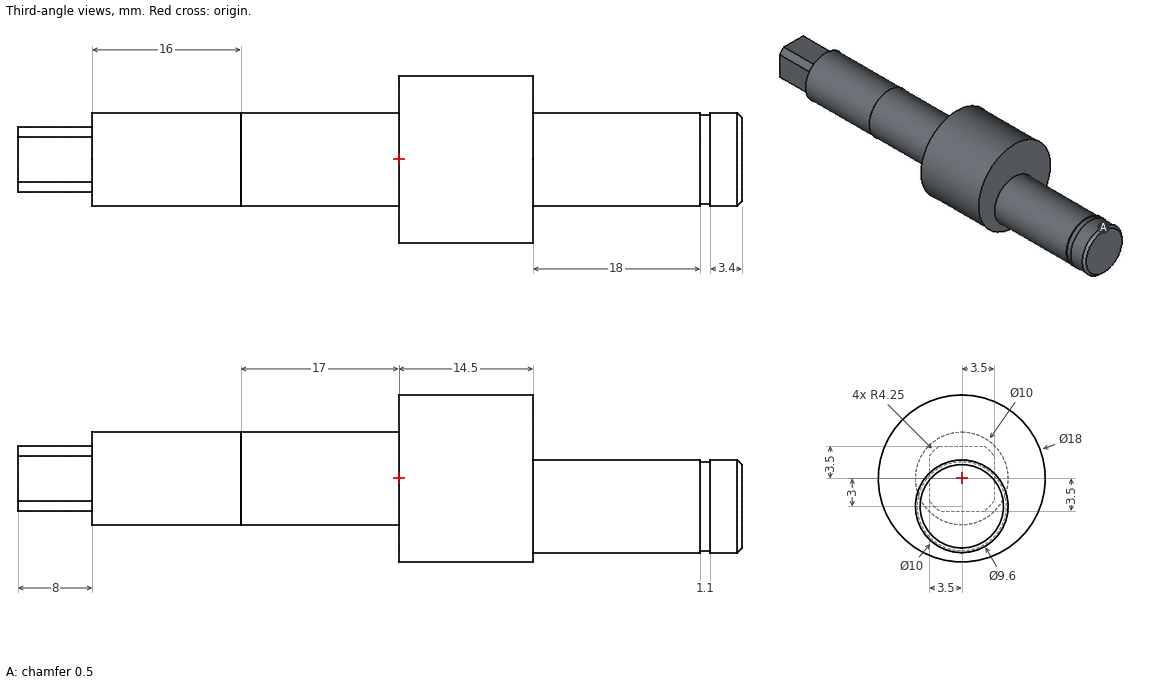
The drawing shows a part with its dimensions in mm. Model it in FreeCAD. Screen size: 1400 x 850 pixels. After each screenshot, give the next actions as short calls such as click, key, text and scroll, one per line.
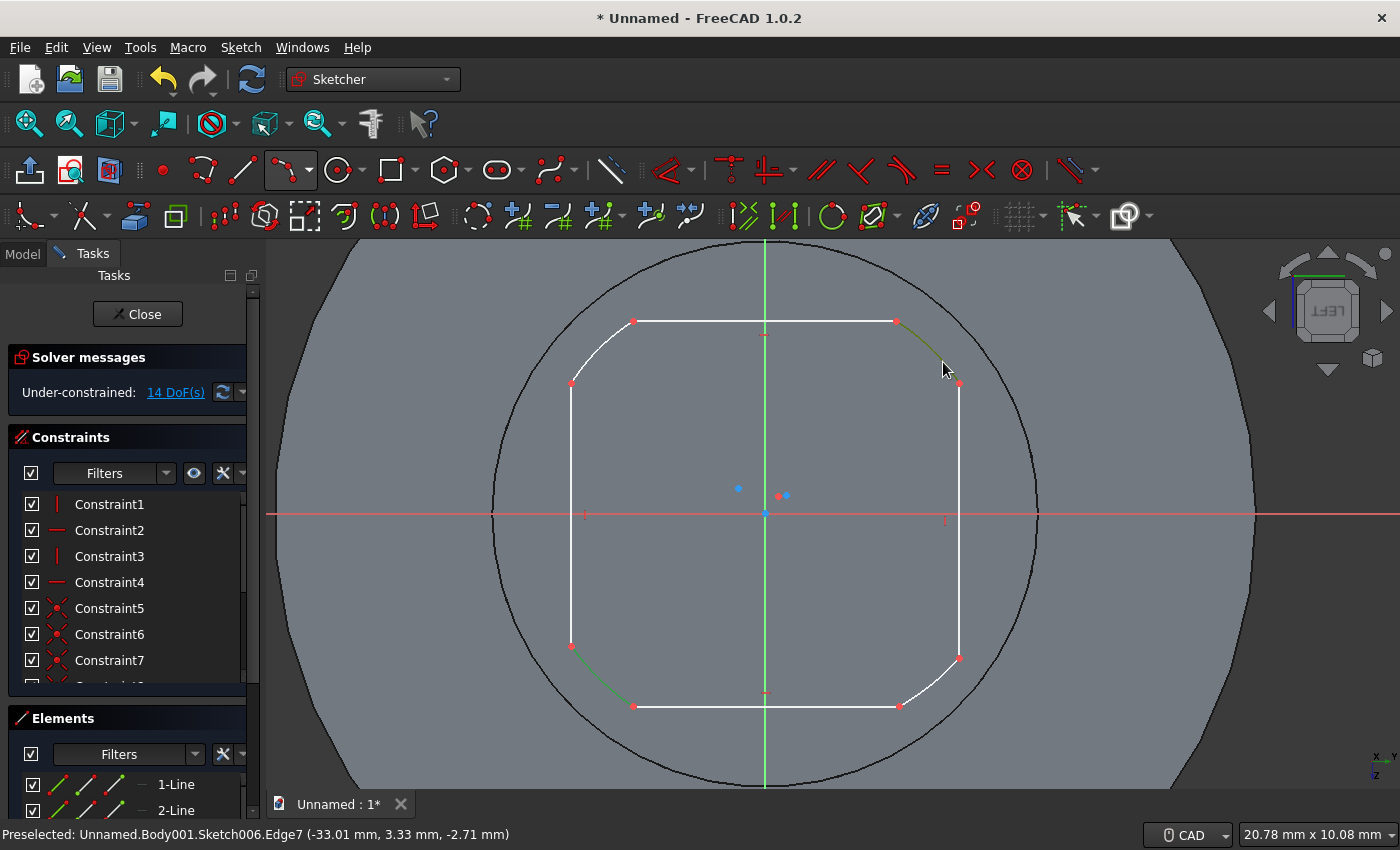
click(730, 170)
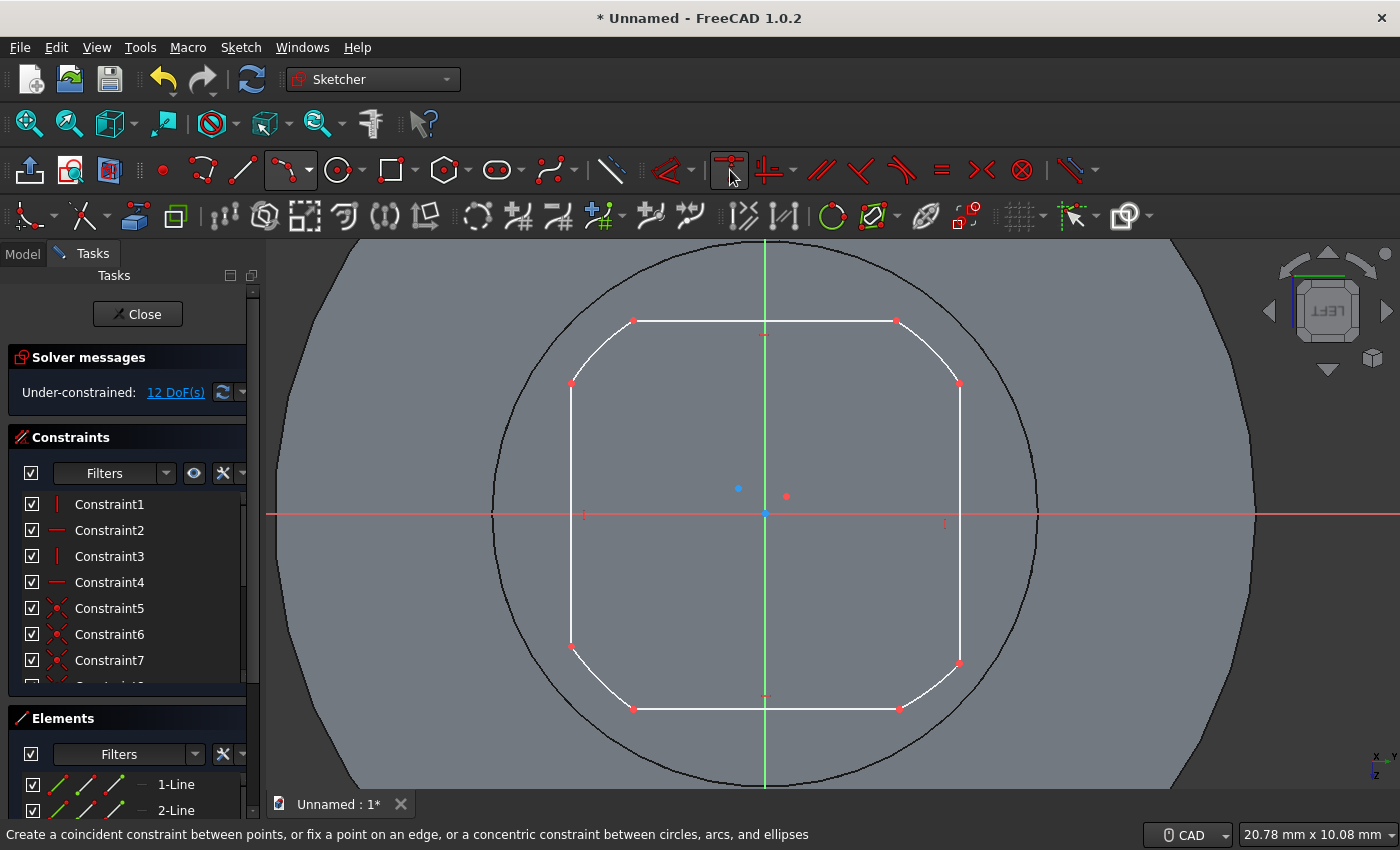
click(588, 667)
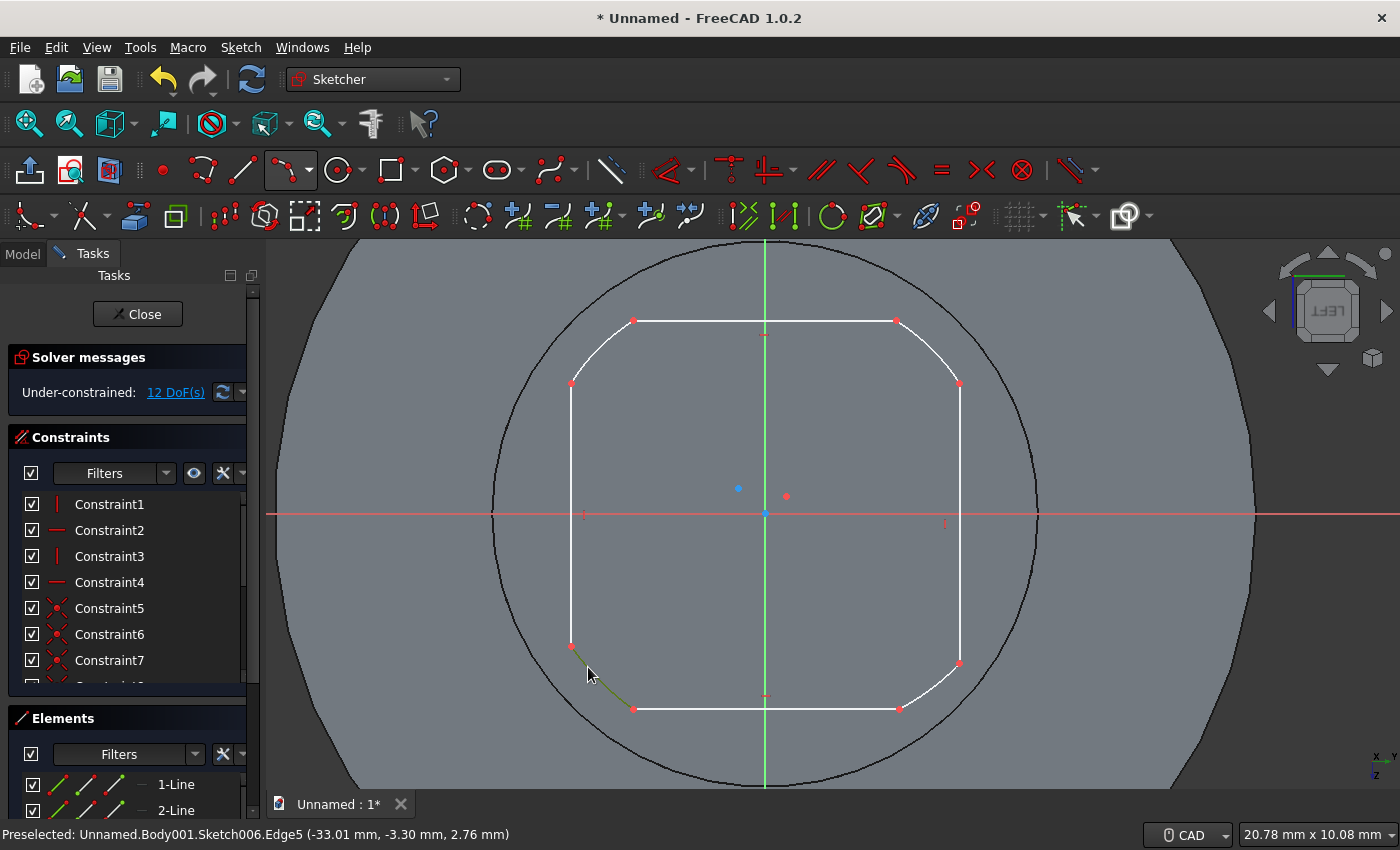
click(612, 337)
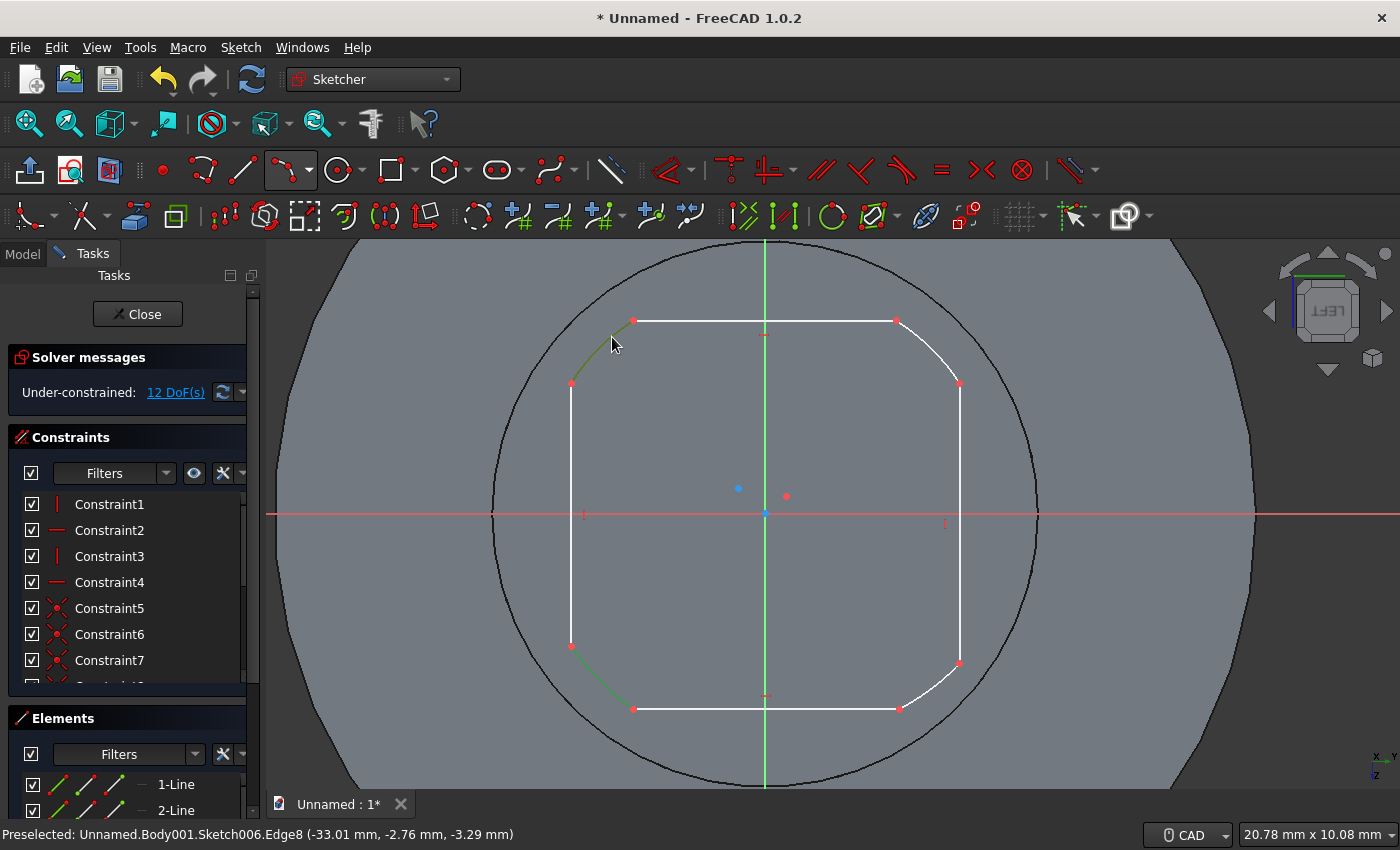
click(730, 170)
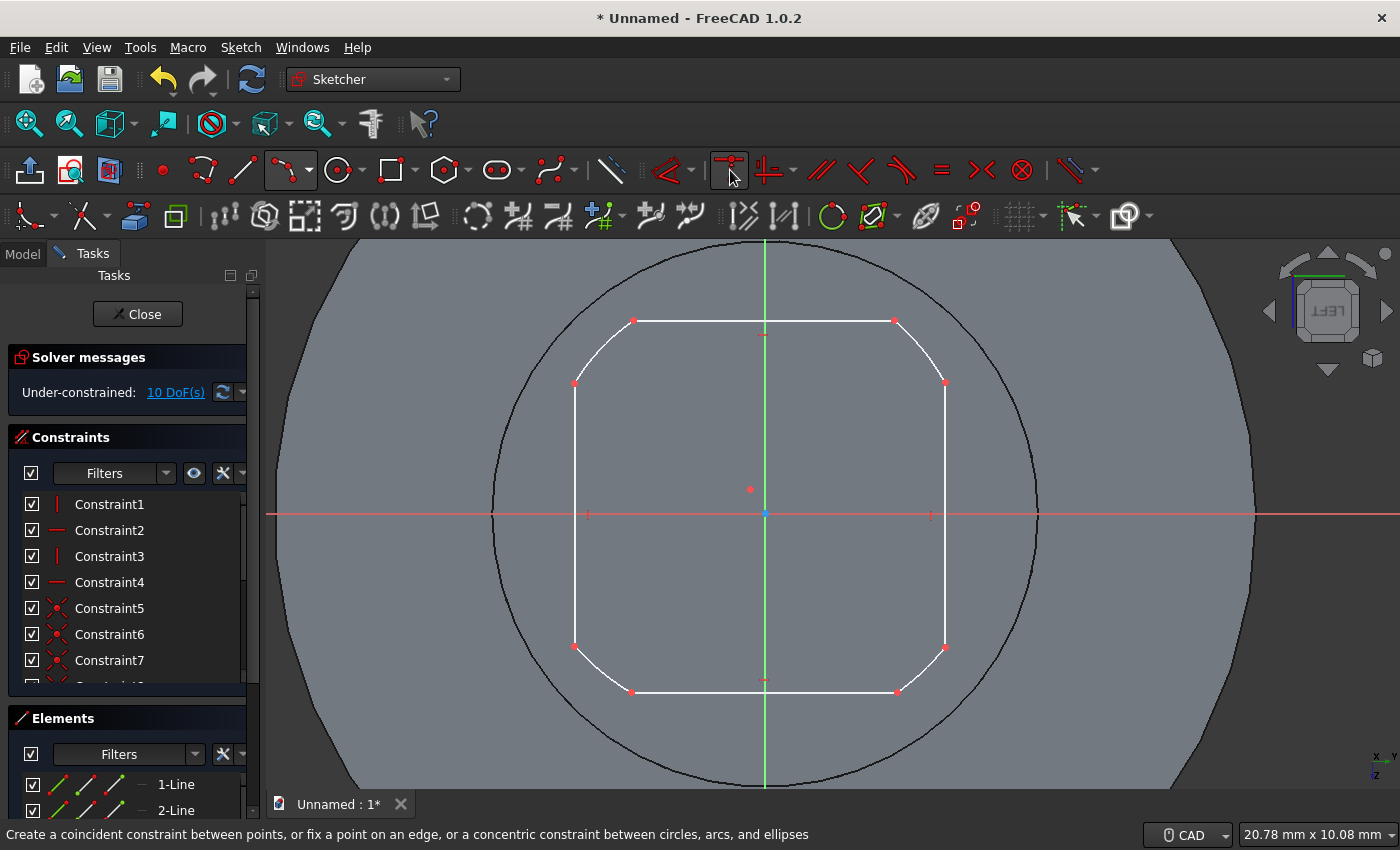
drag(741, 480, 775, 524)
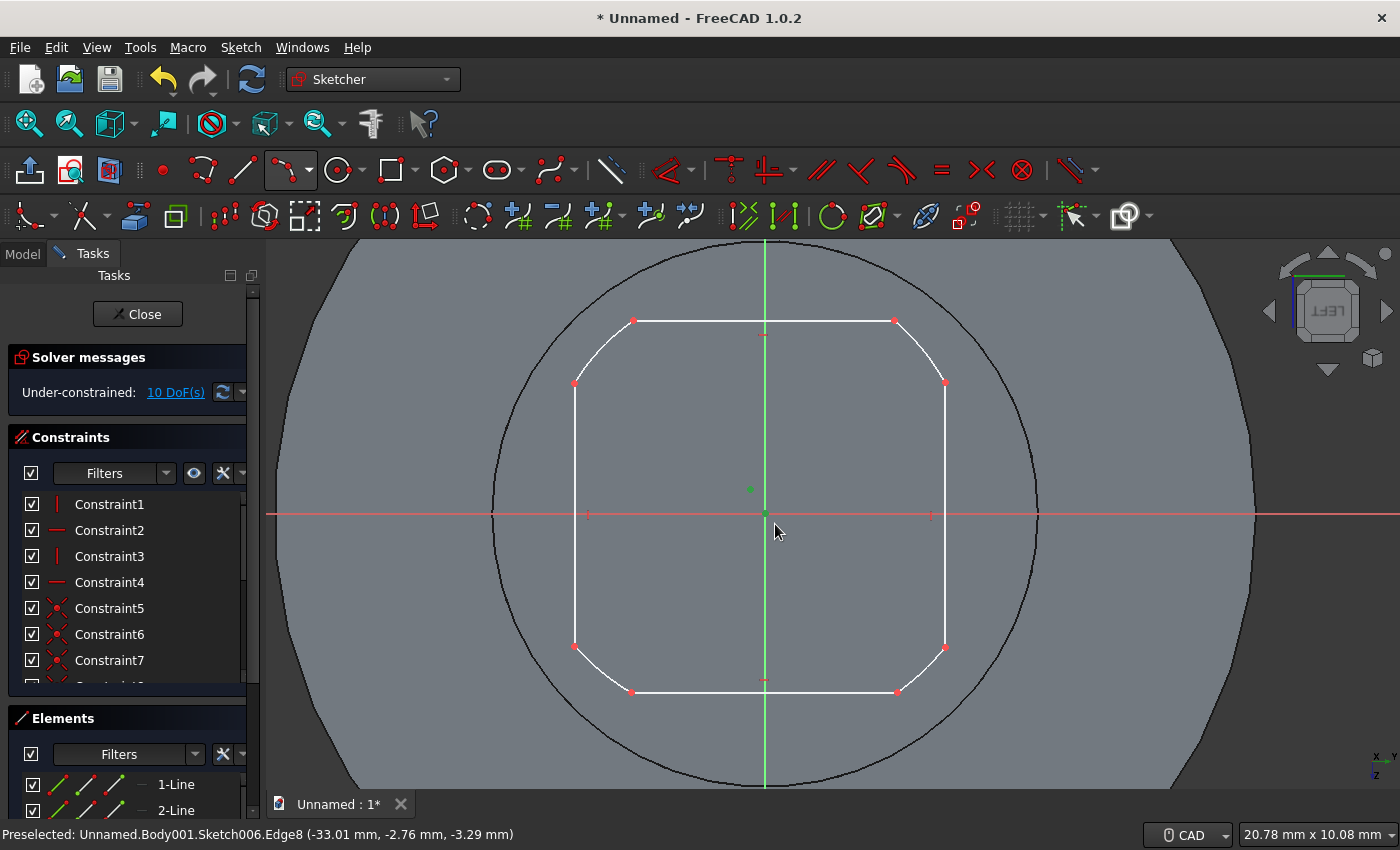
click(730, 170)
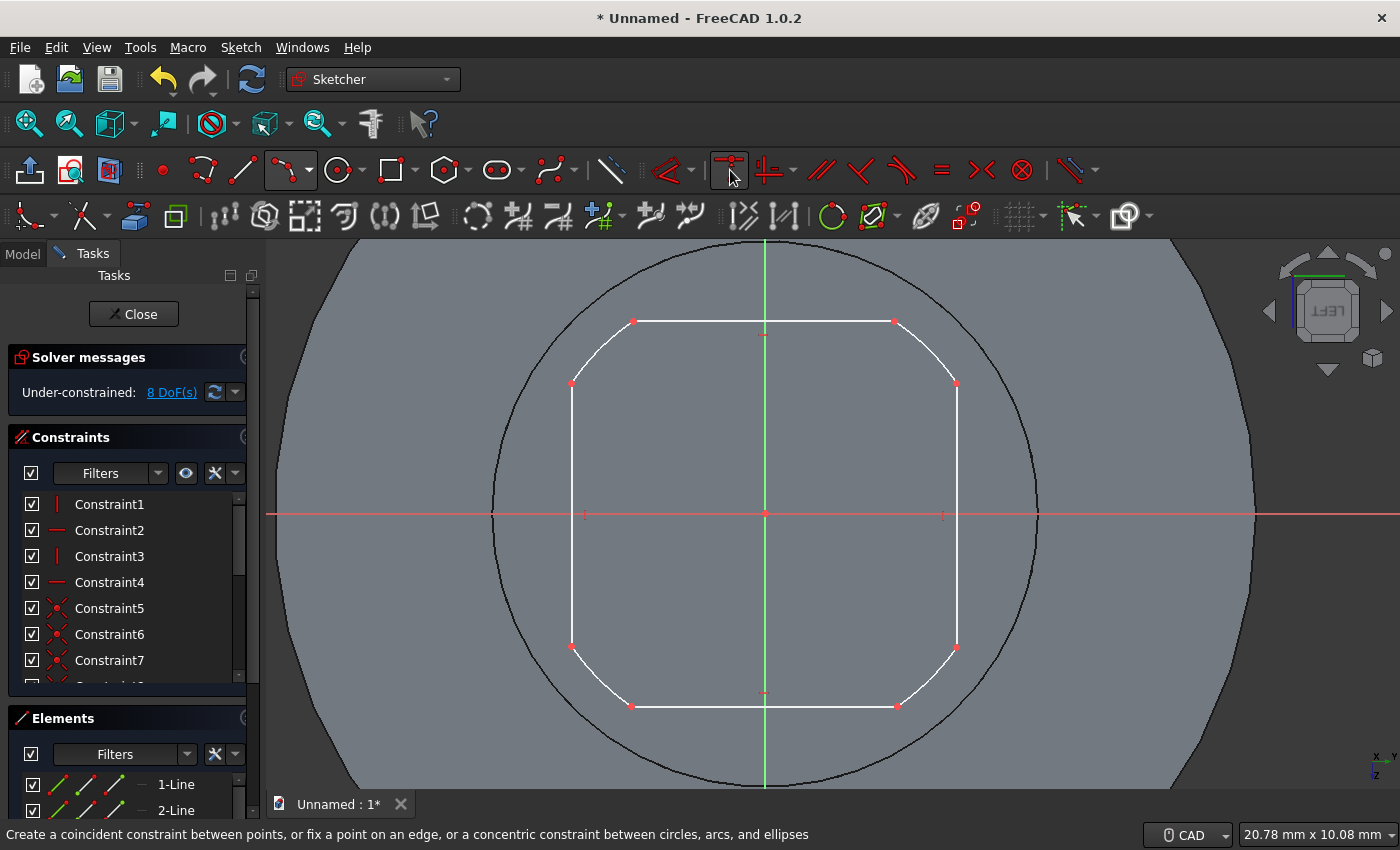
click(587, 667)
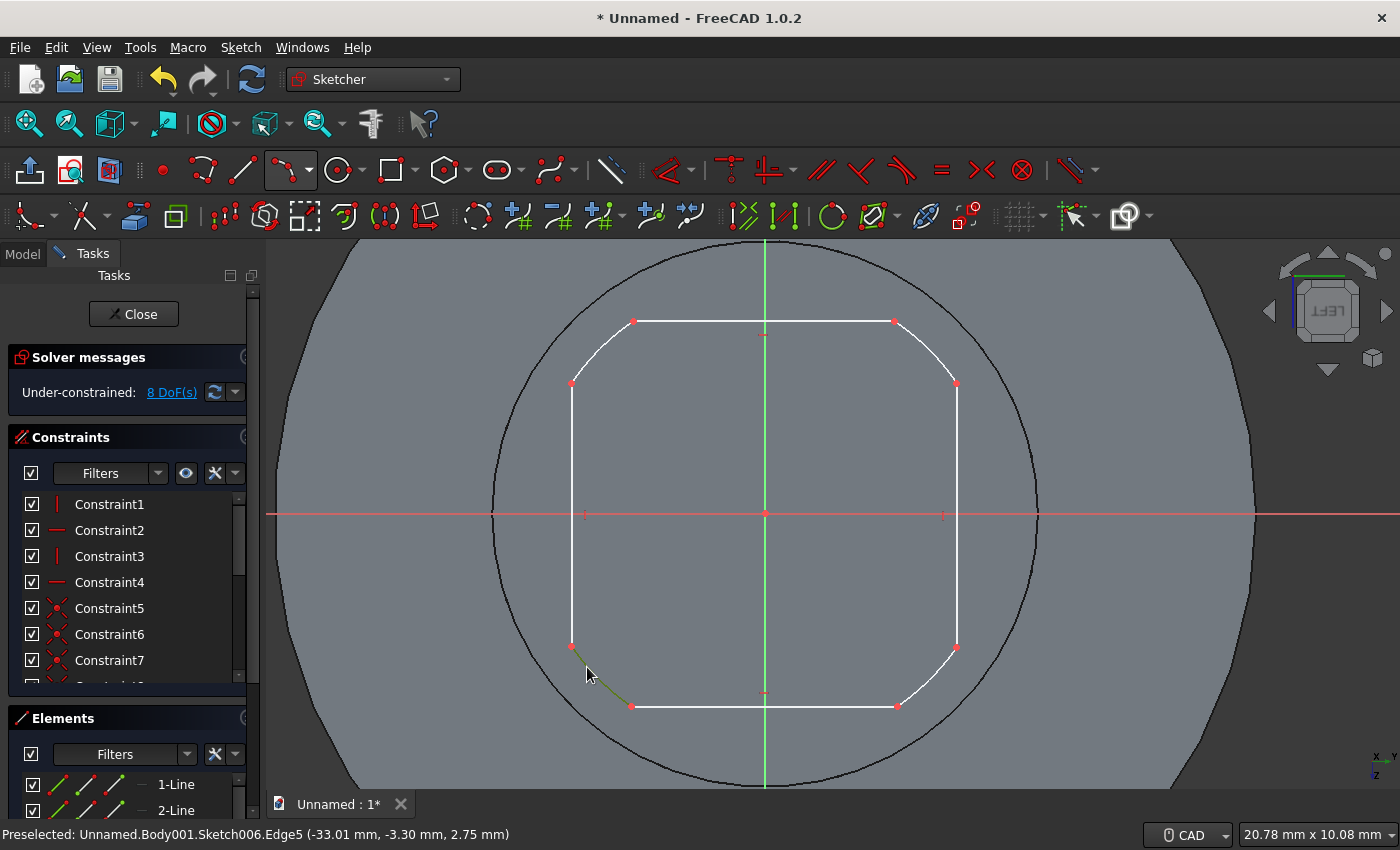
click(917, 691)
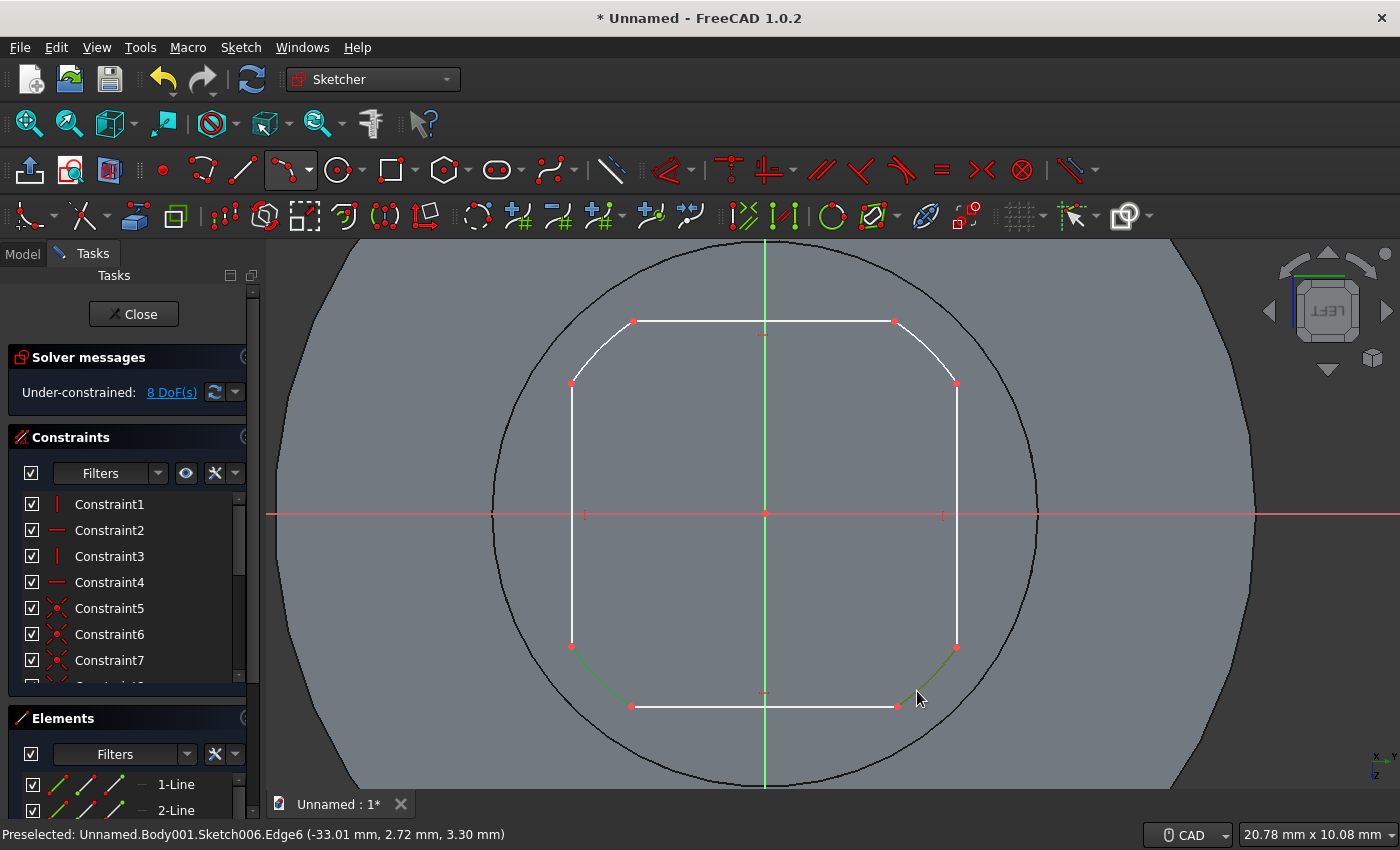
click(941, 362)